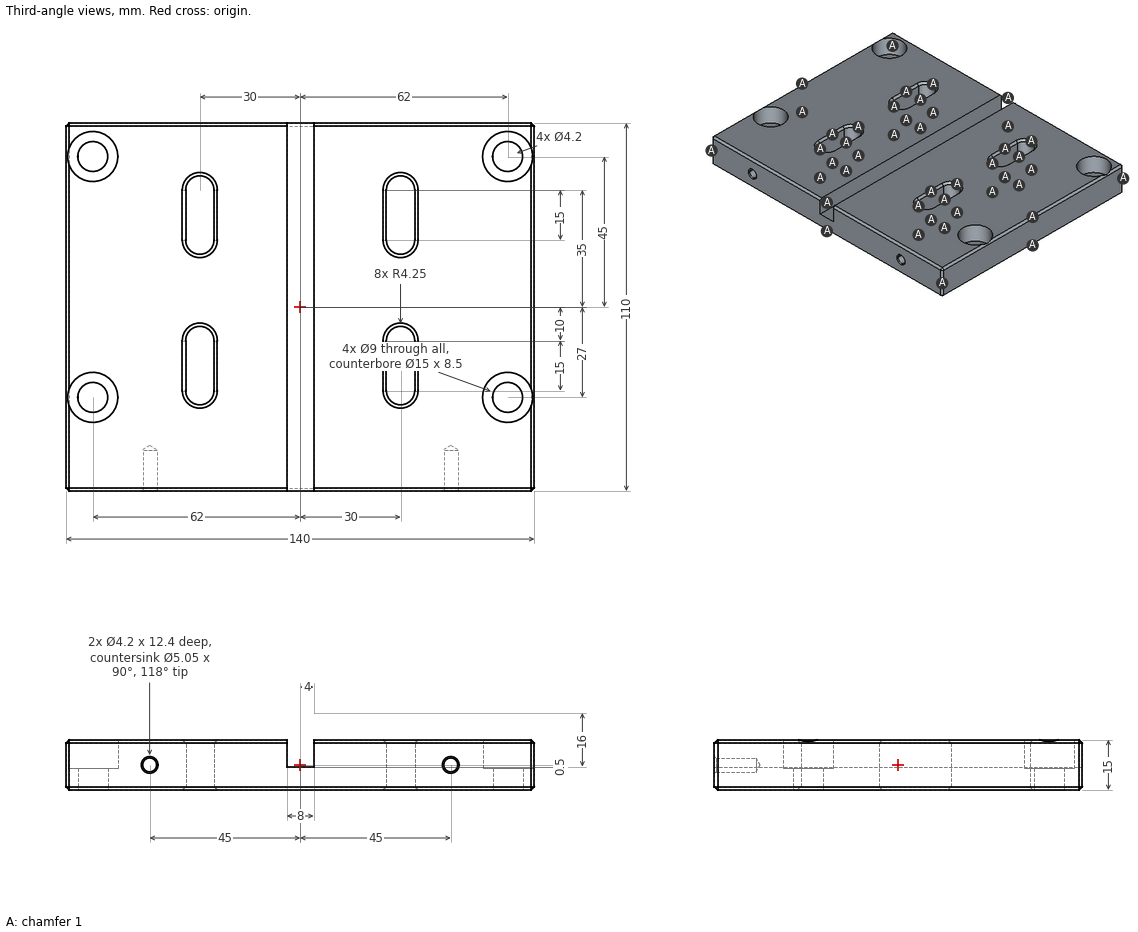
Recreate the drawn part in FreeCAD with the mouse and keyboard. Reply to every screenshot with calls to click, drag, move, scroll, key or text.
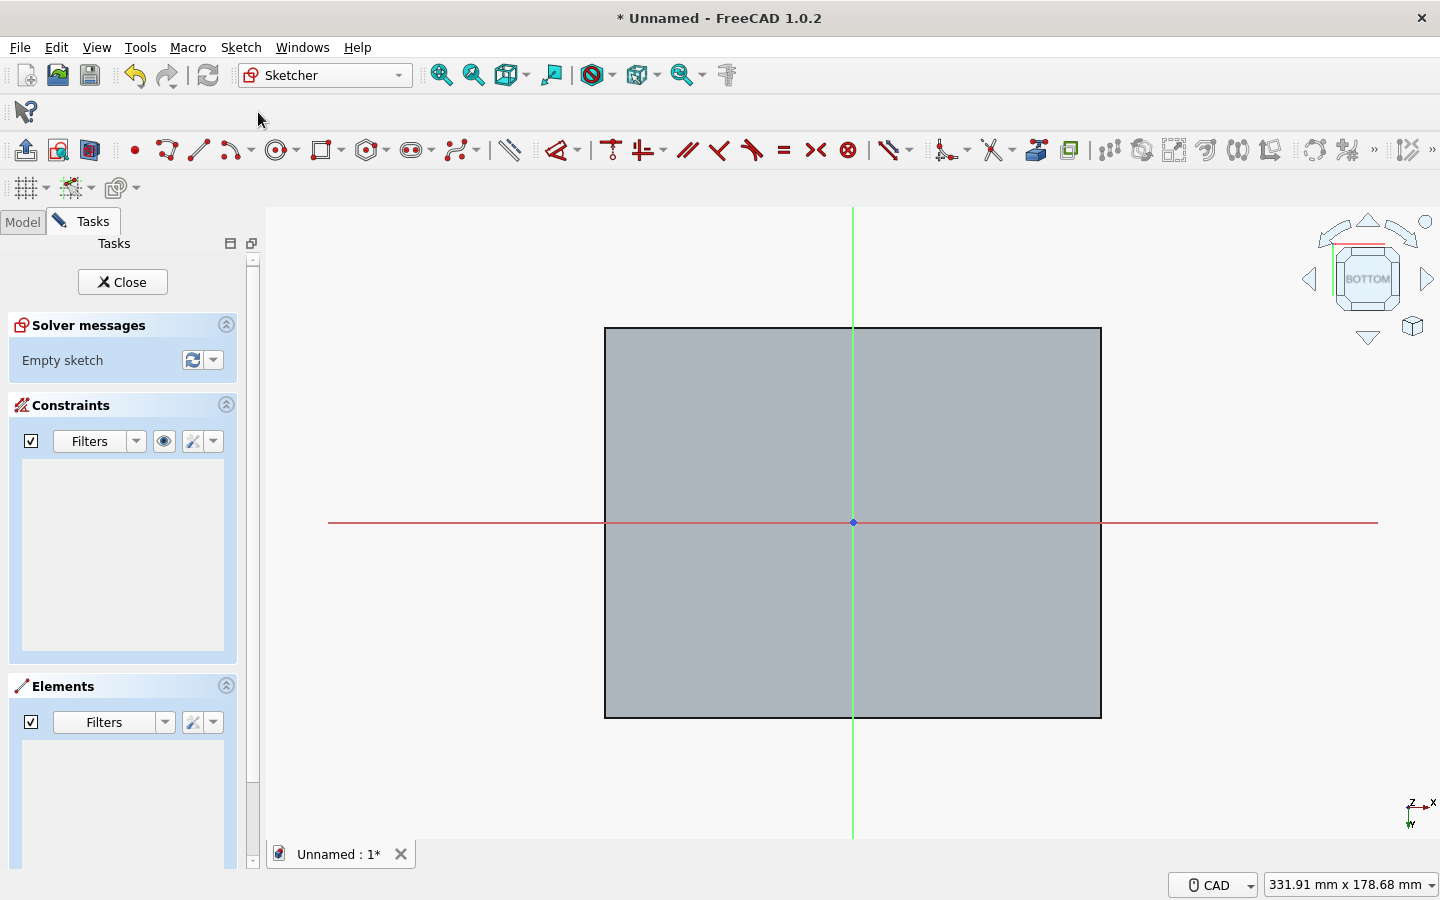
scroll(936, 562, up, 3)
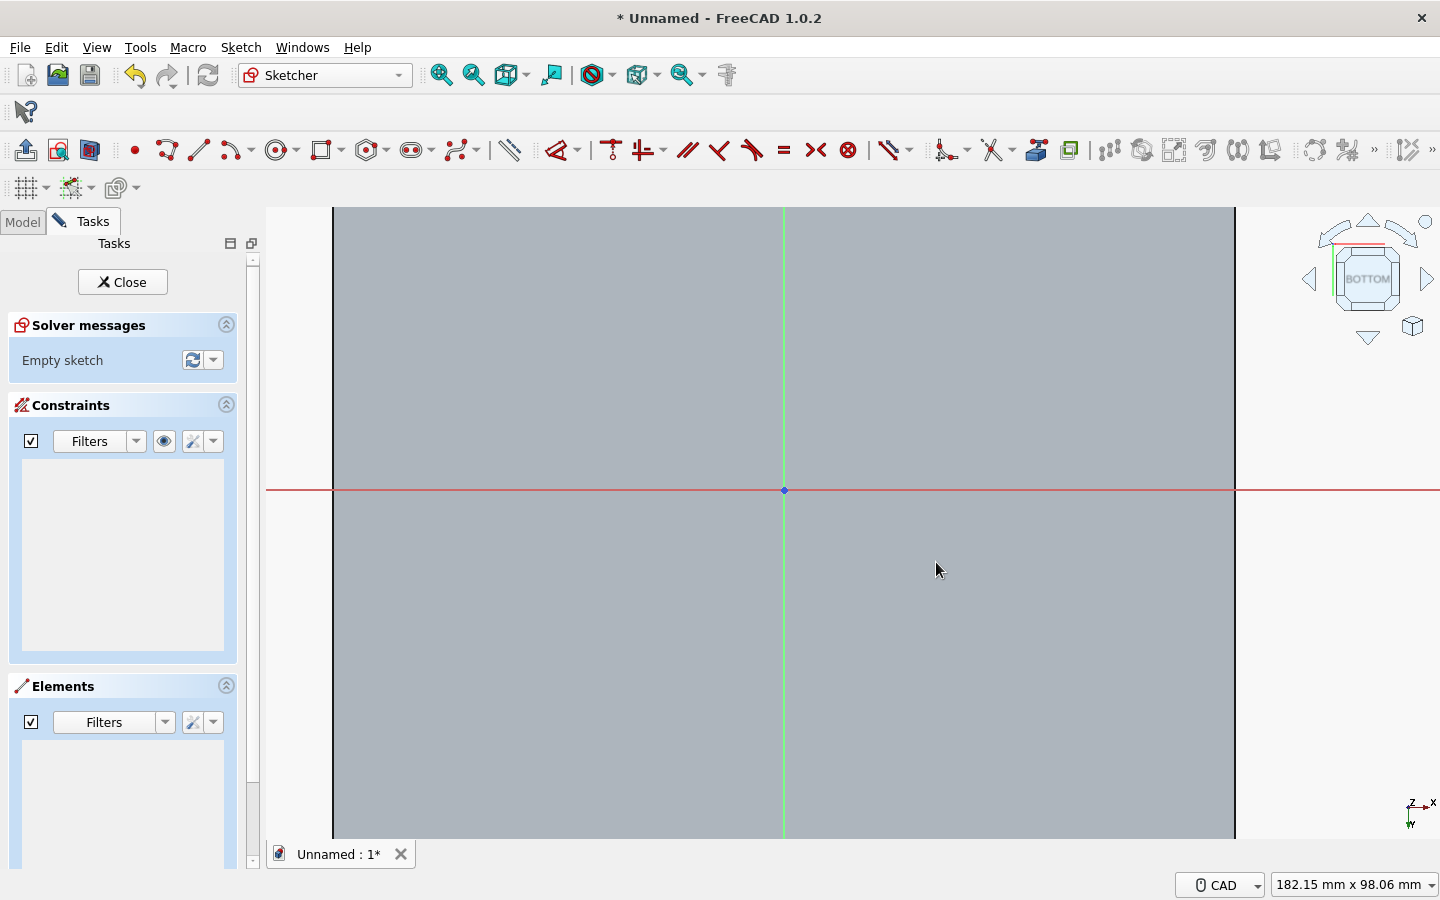
click(412, 150)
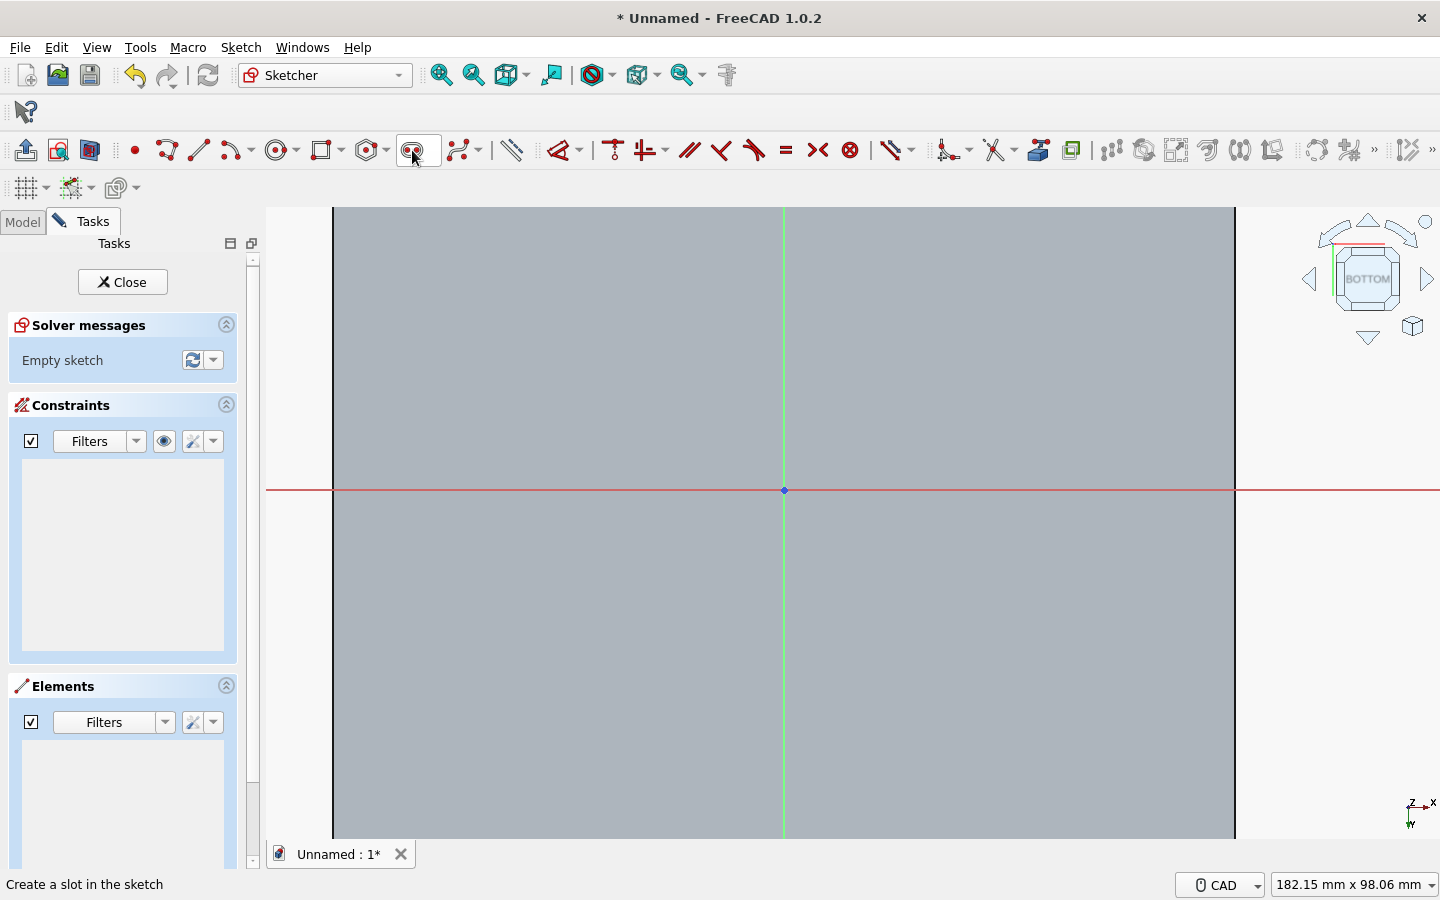
click(978, 426)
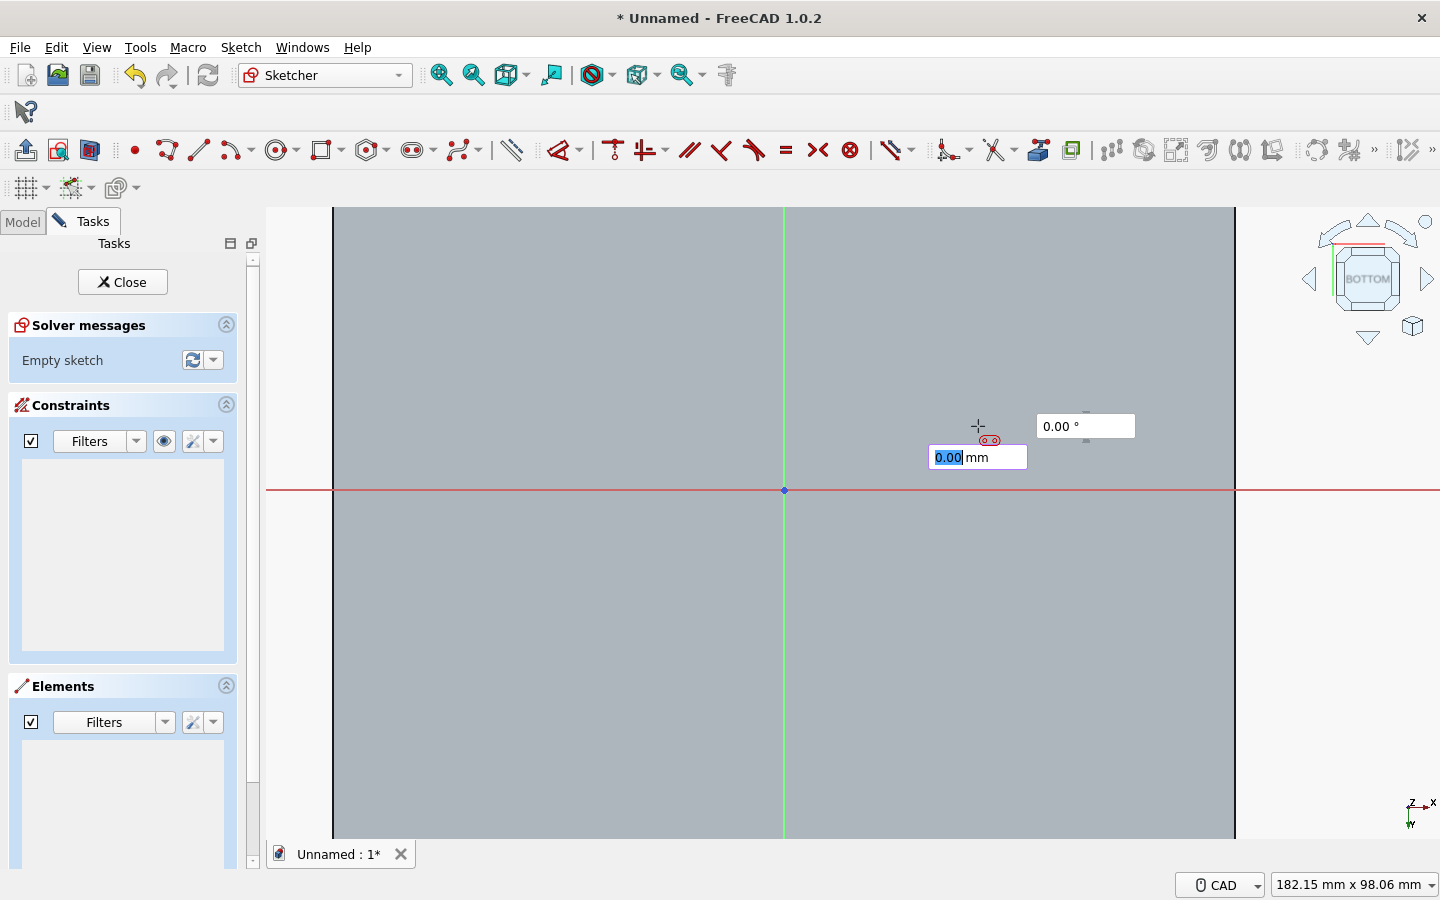
click(978, 329)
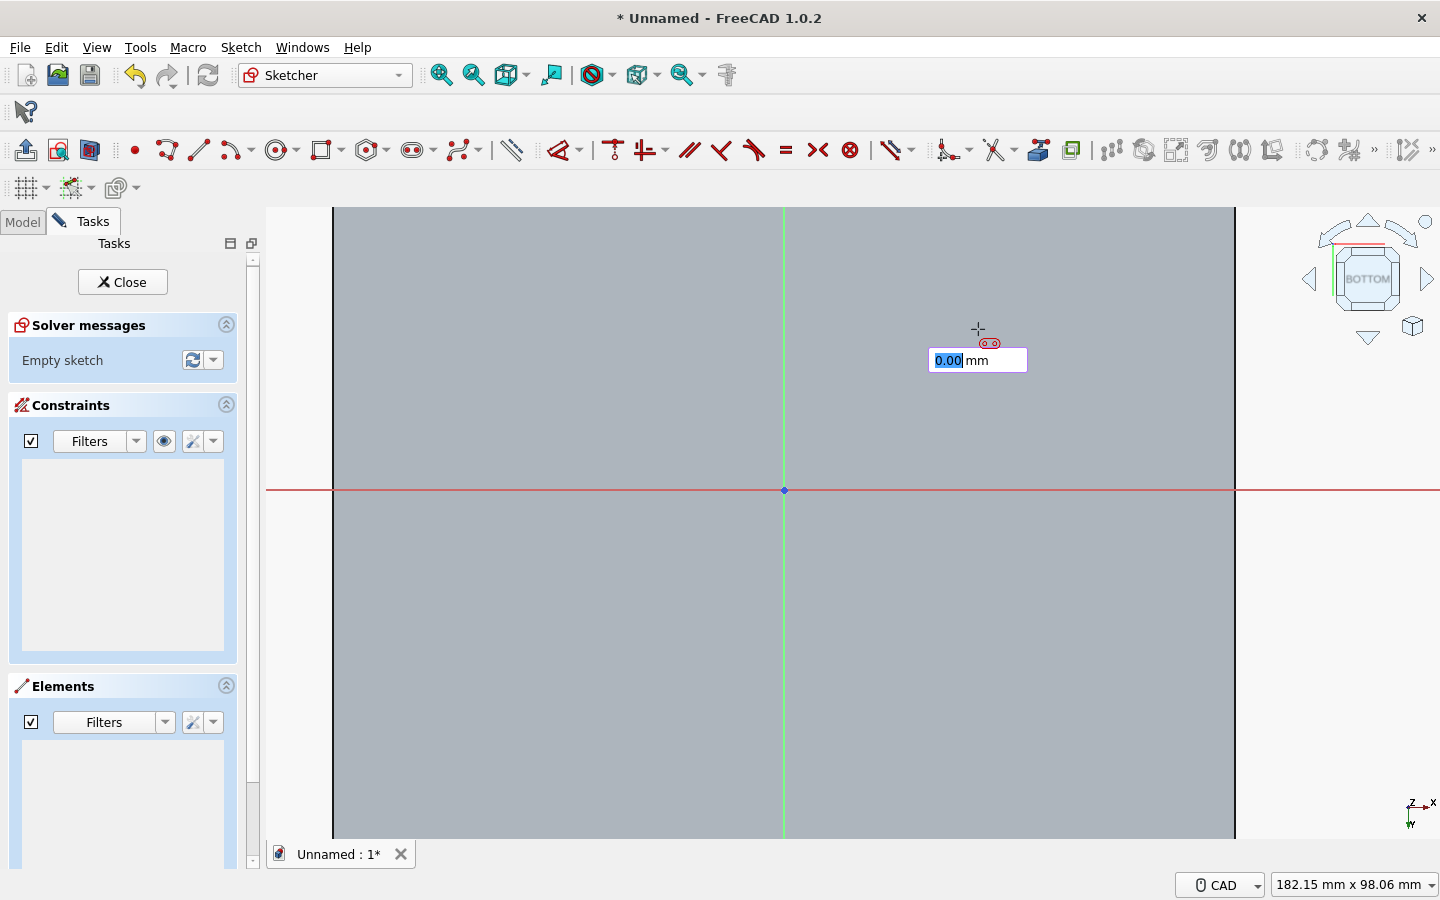
click(950, 378)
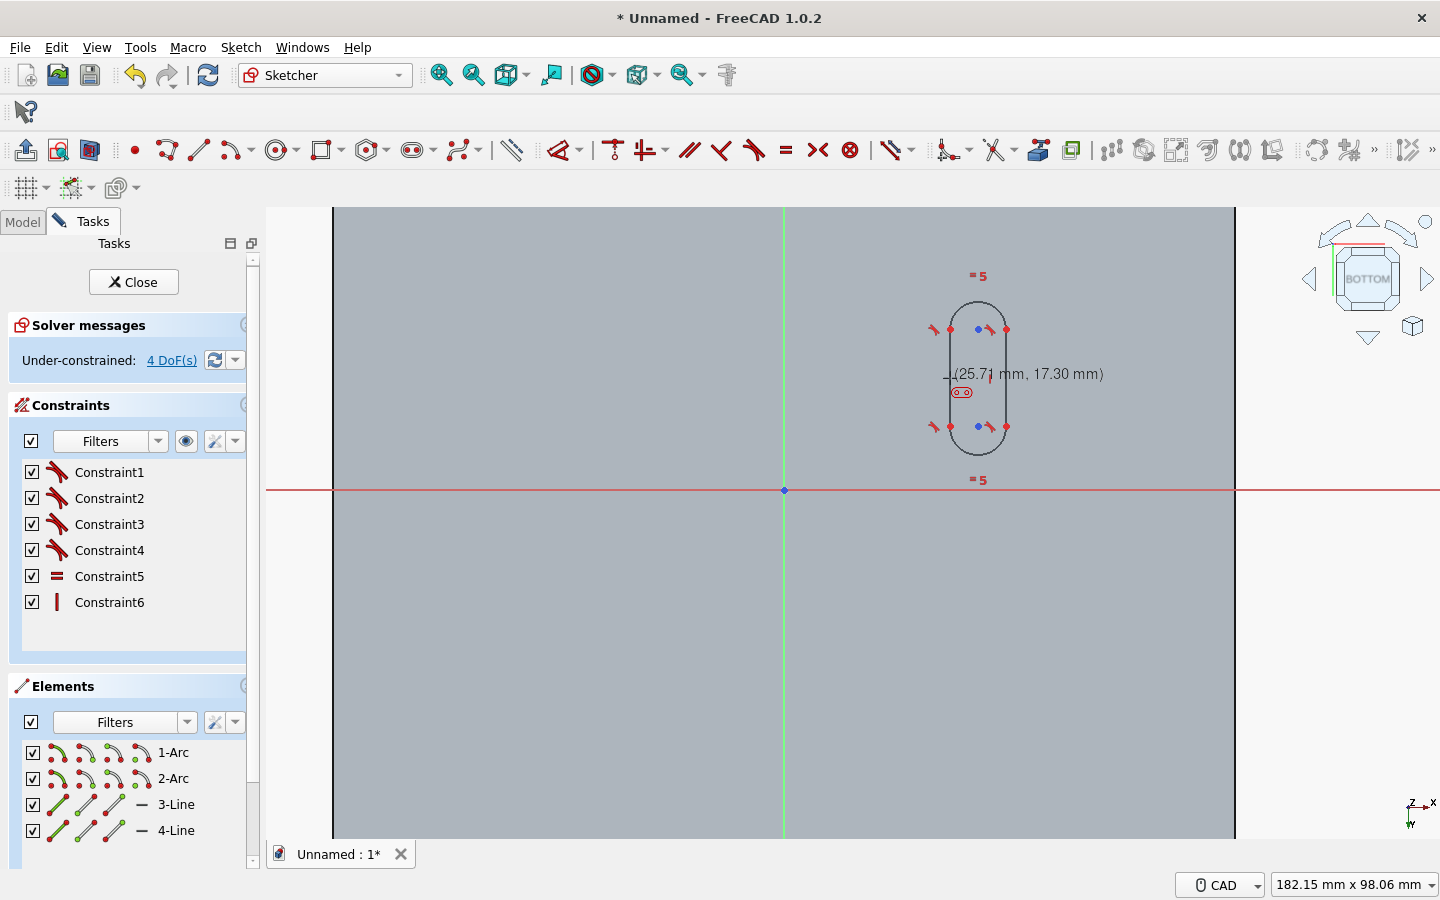
click(978, 716)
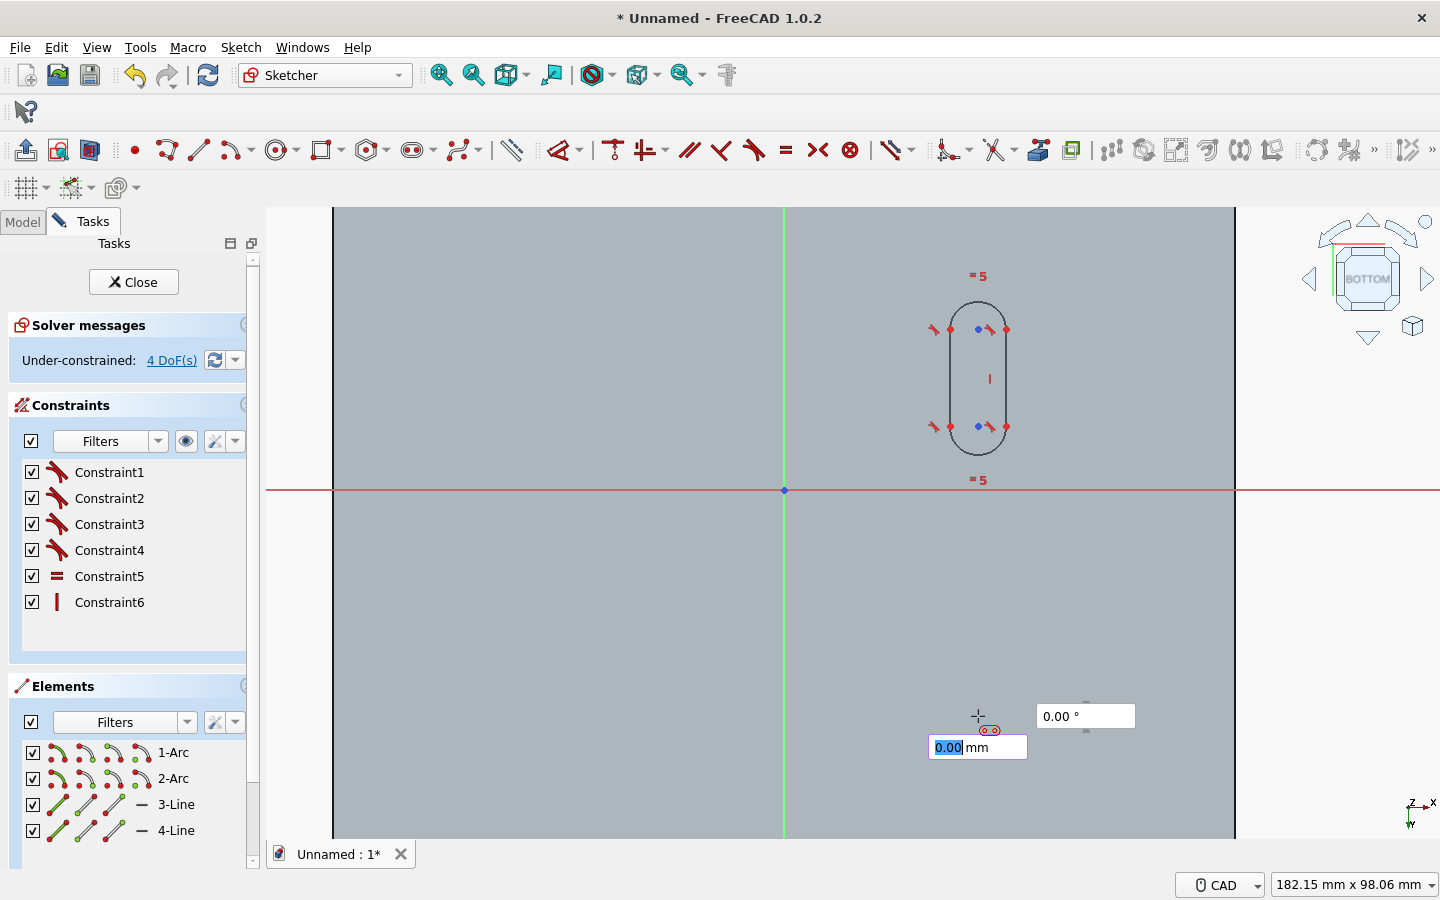
click(978, 619)